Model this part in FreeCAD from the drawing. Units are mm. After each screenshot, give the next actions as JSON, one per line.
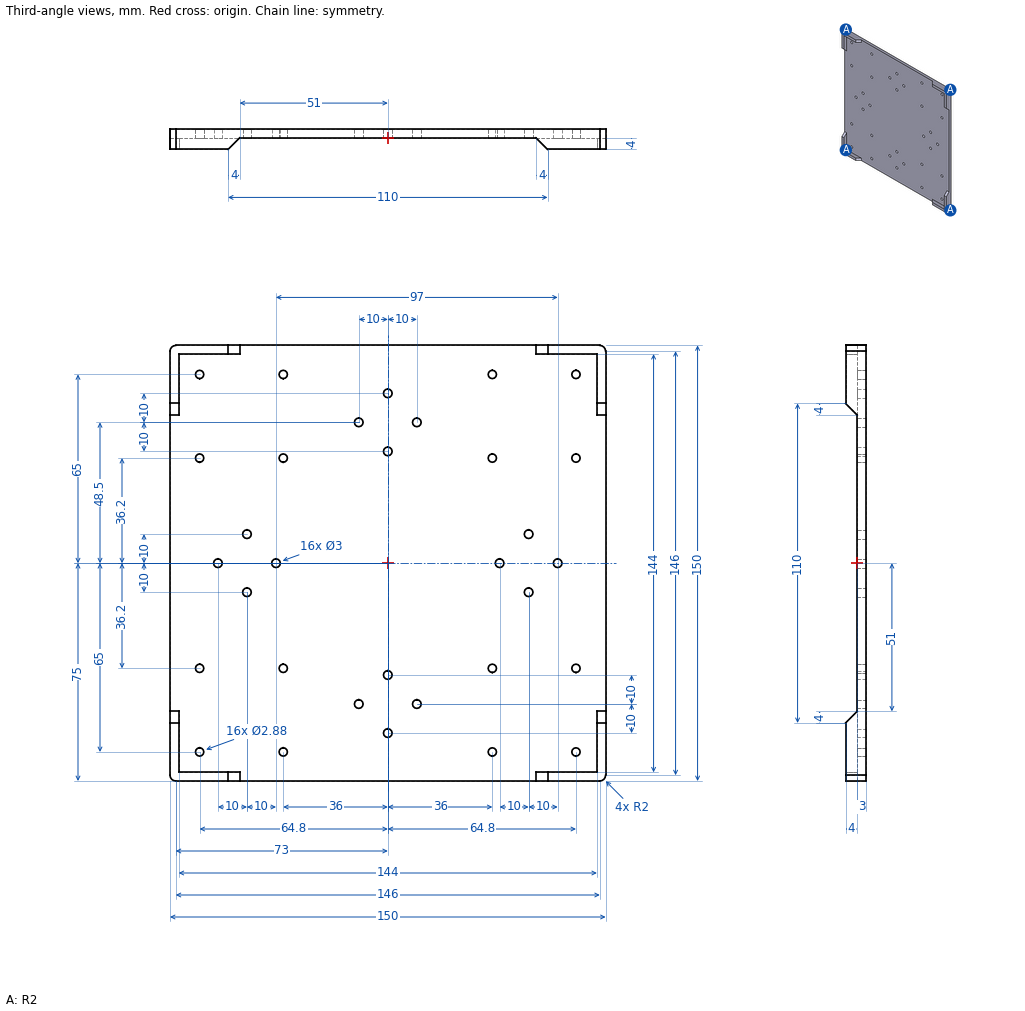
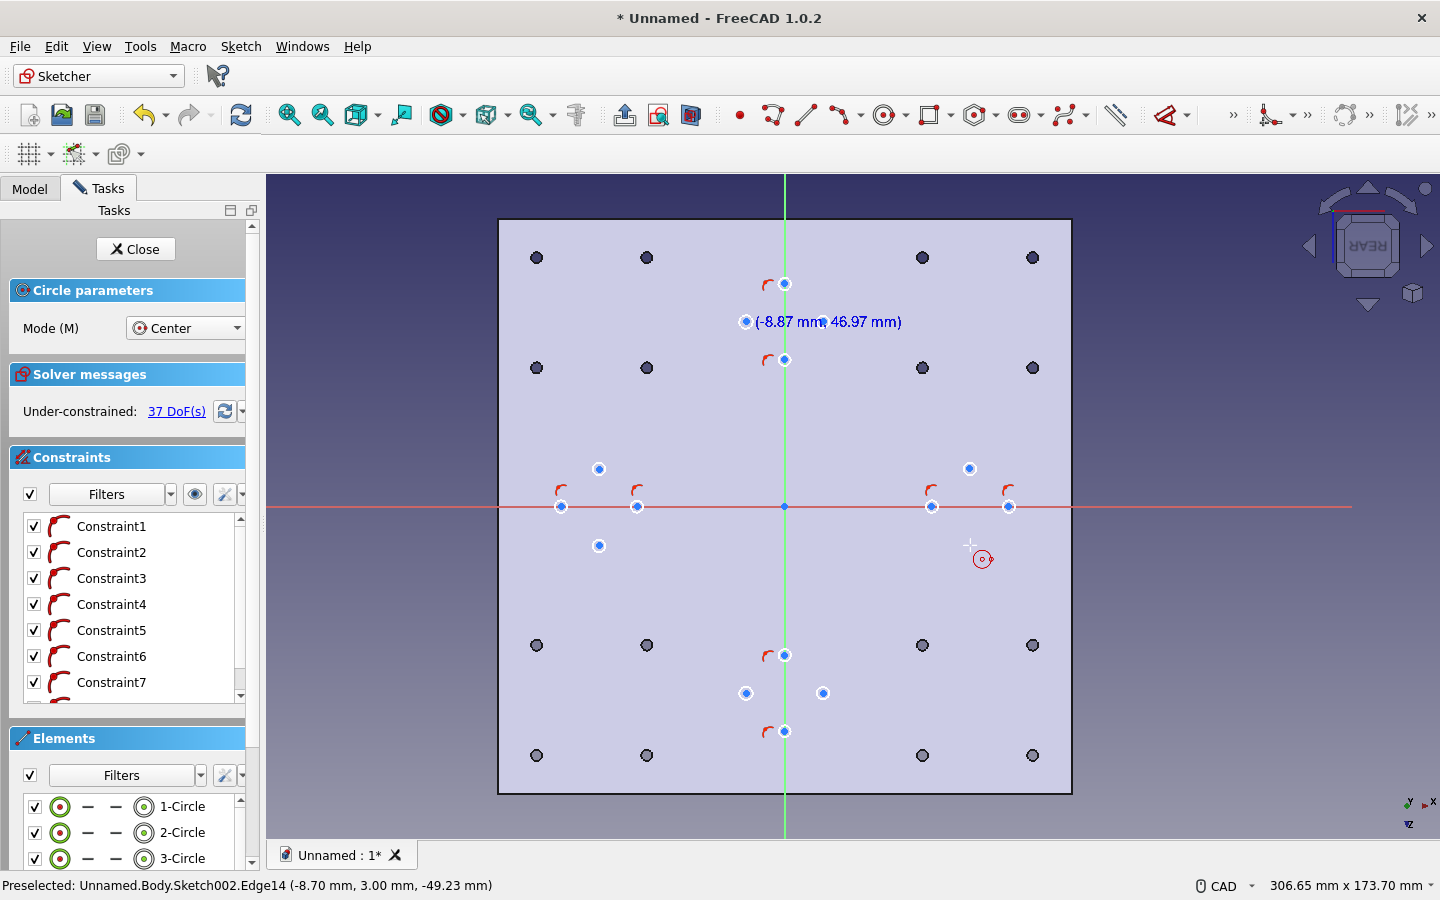
{"action": "left_click", "coordinate": [970, 545]}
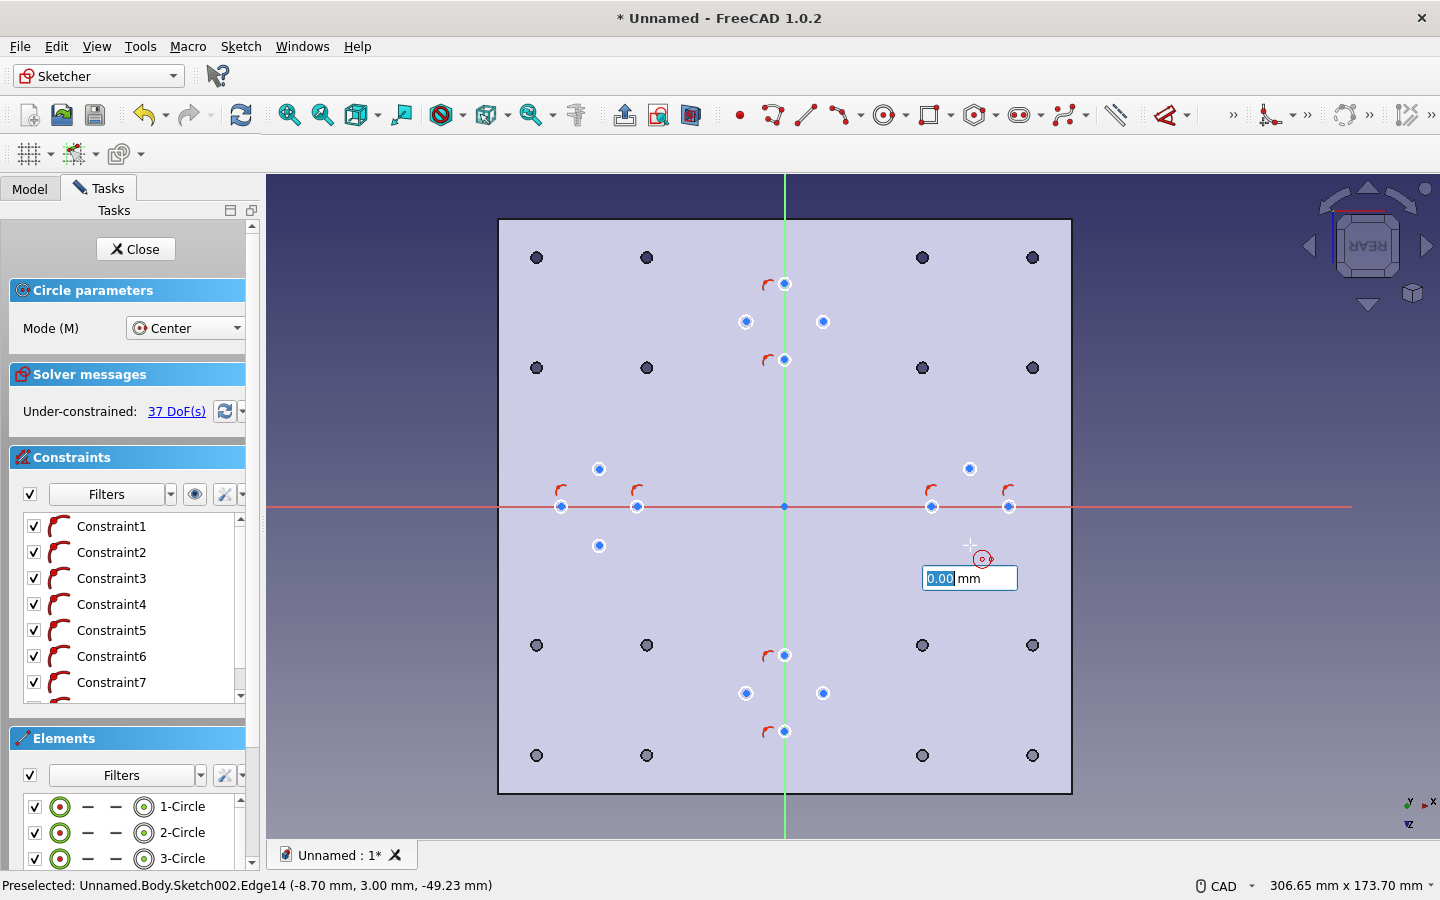
{"action": "scroll", "coordinate": [974, 541], "scroll_direction": "up", "scroll_amount": 6}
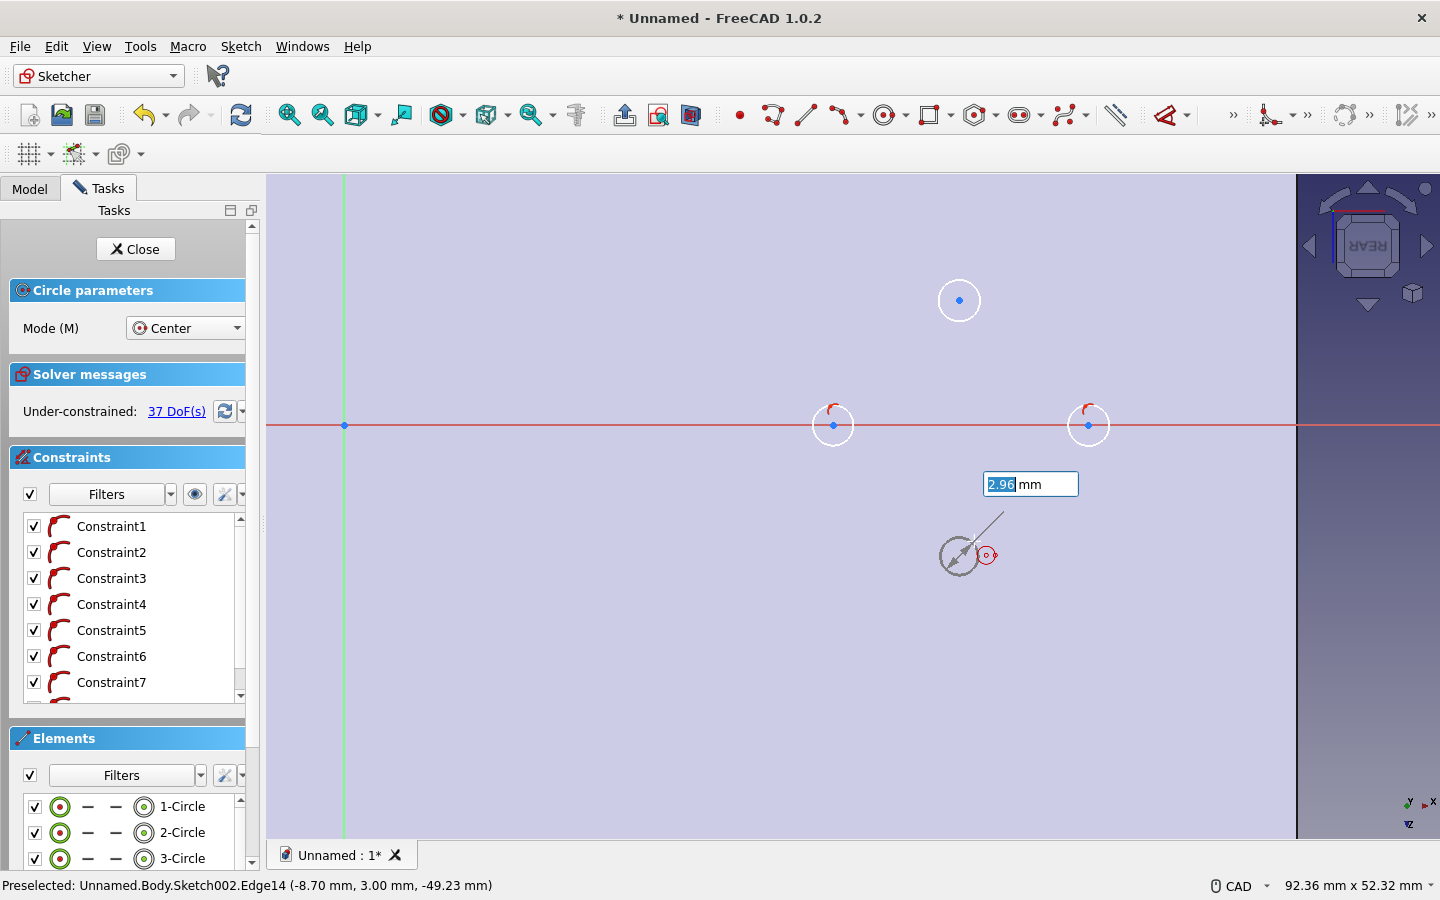
{"action": "left_click", "coordinate": [974, 539]}
{"action": "key", "text": "Escape"}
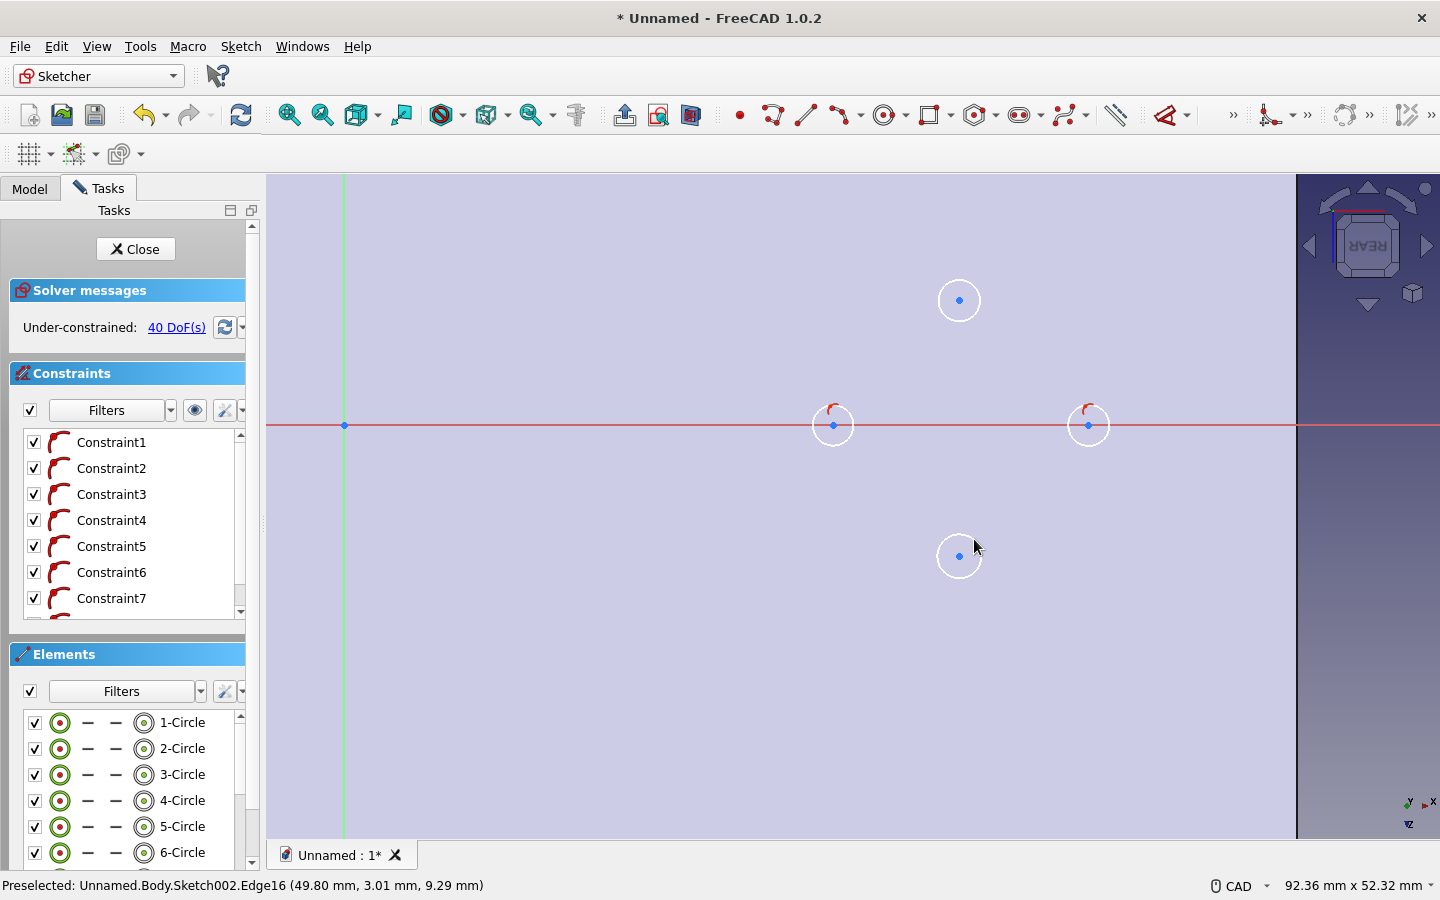
{"action": "scroll", "coordinate": [974, 541], "scroll_direction": "down", "scroll_amount": 6}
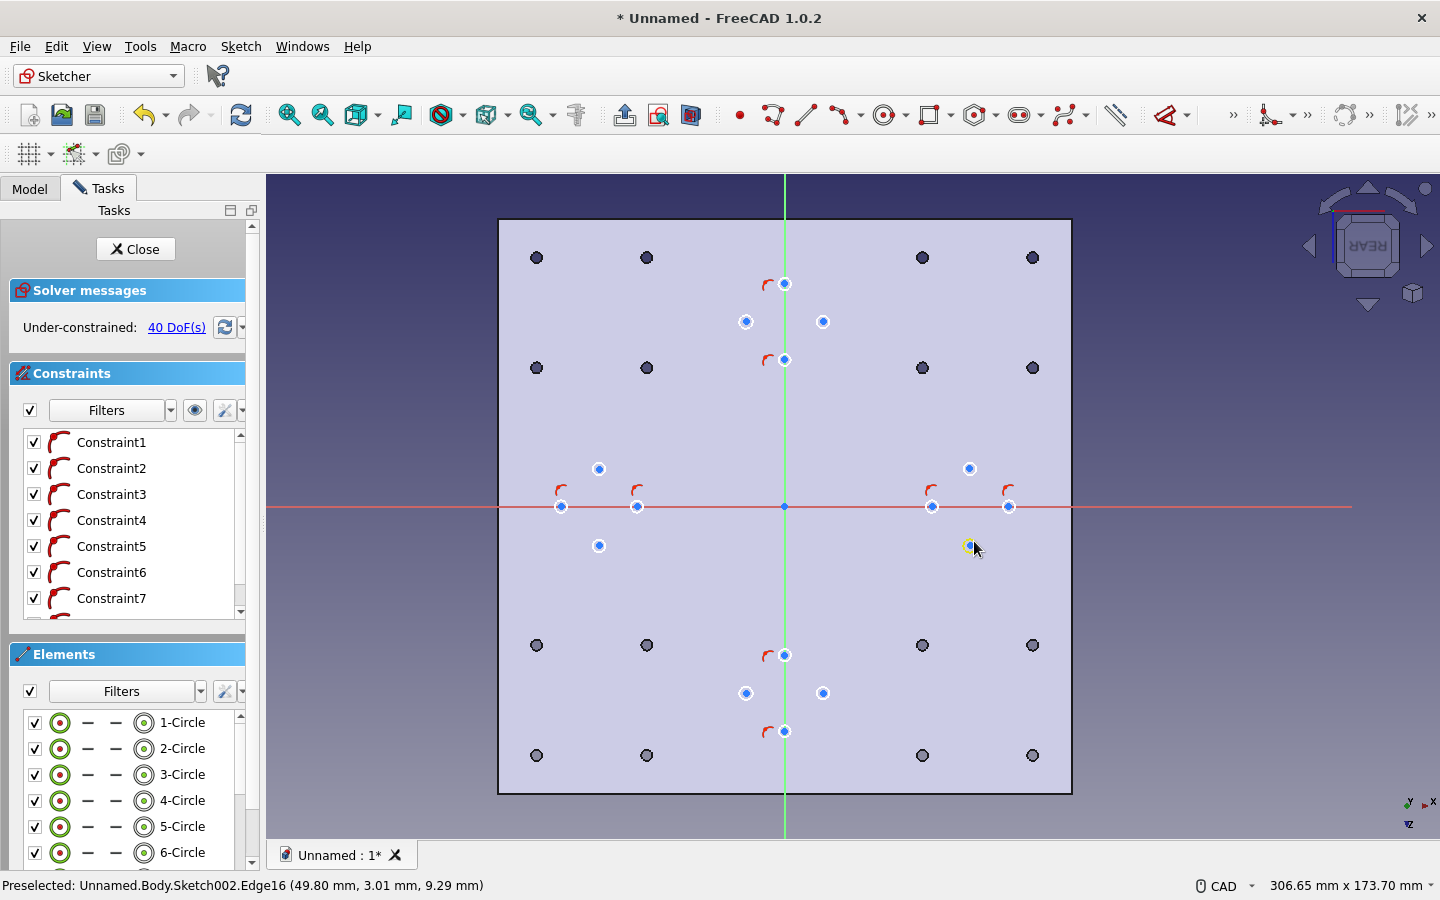
{"action": "scroll", "coordinate": [641, 502], "scroll_direction": "up", "scroll_amount": 6}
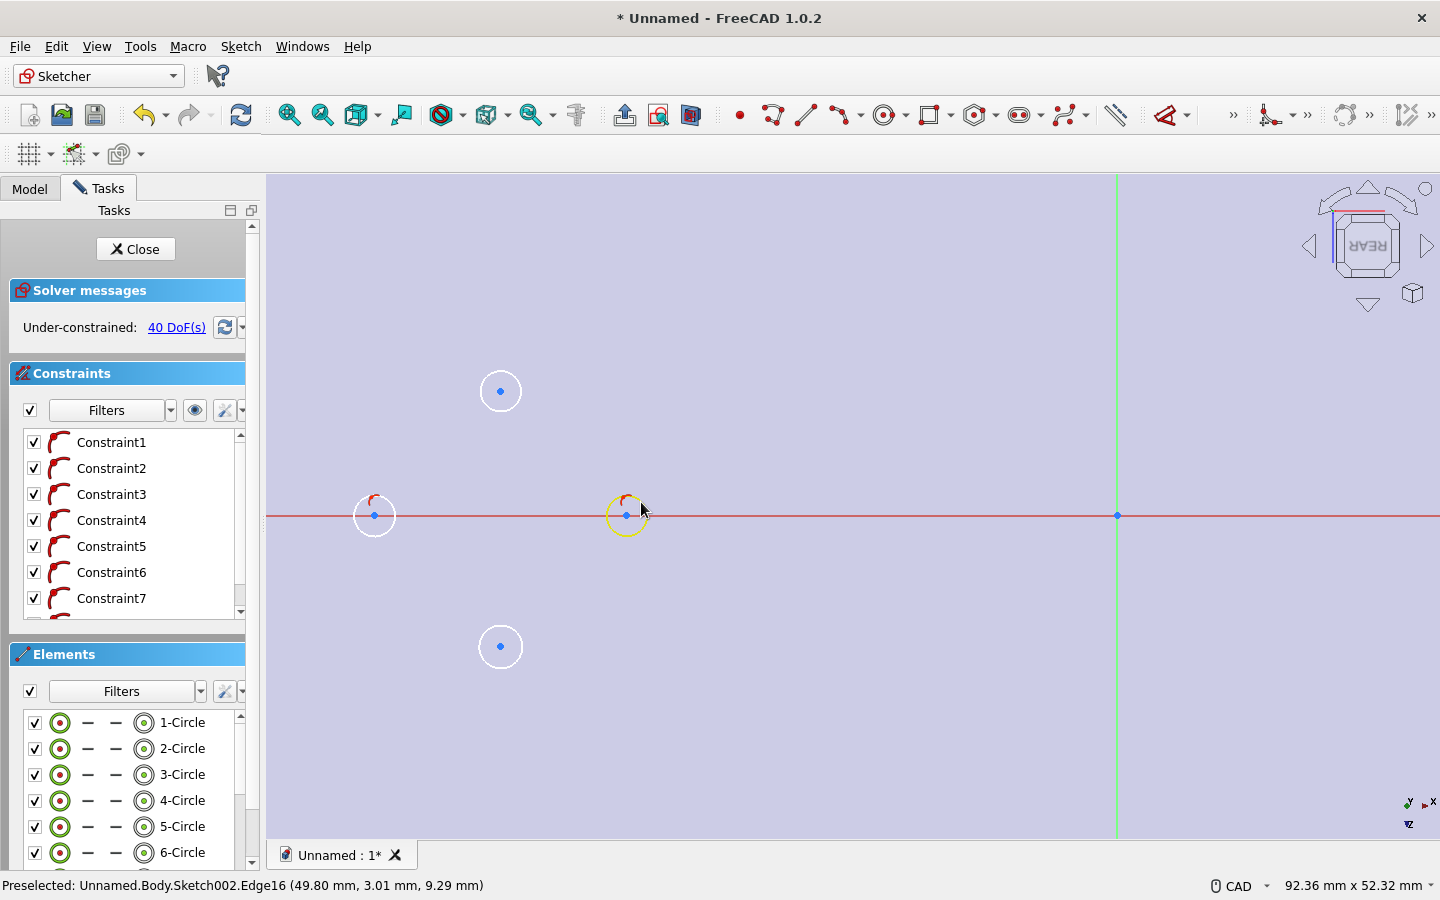
{"action": "left_click", "coordinate": [641, 502]}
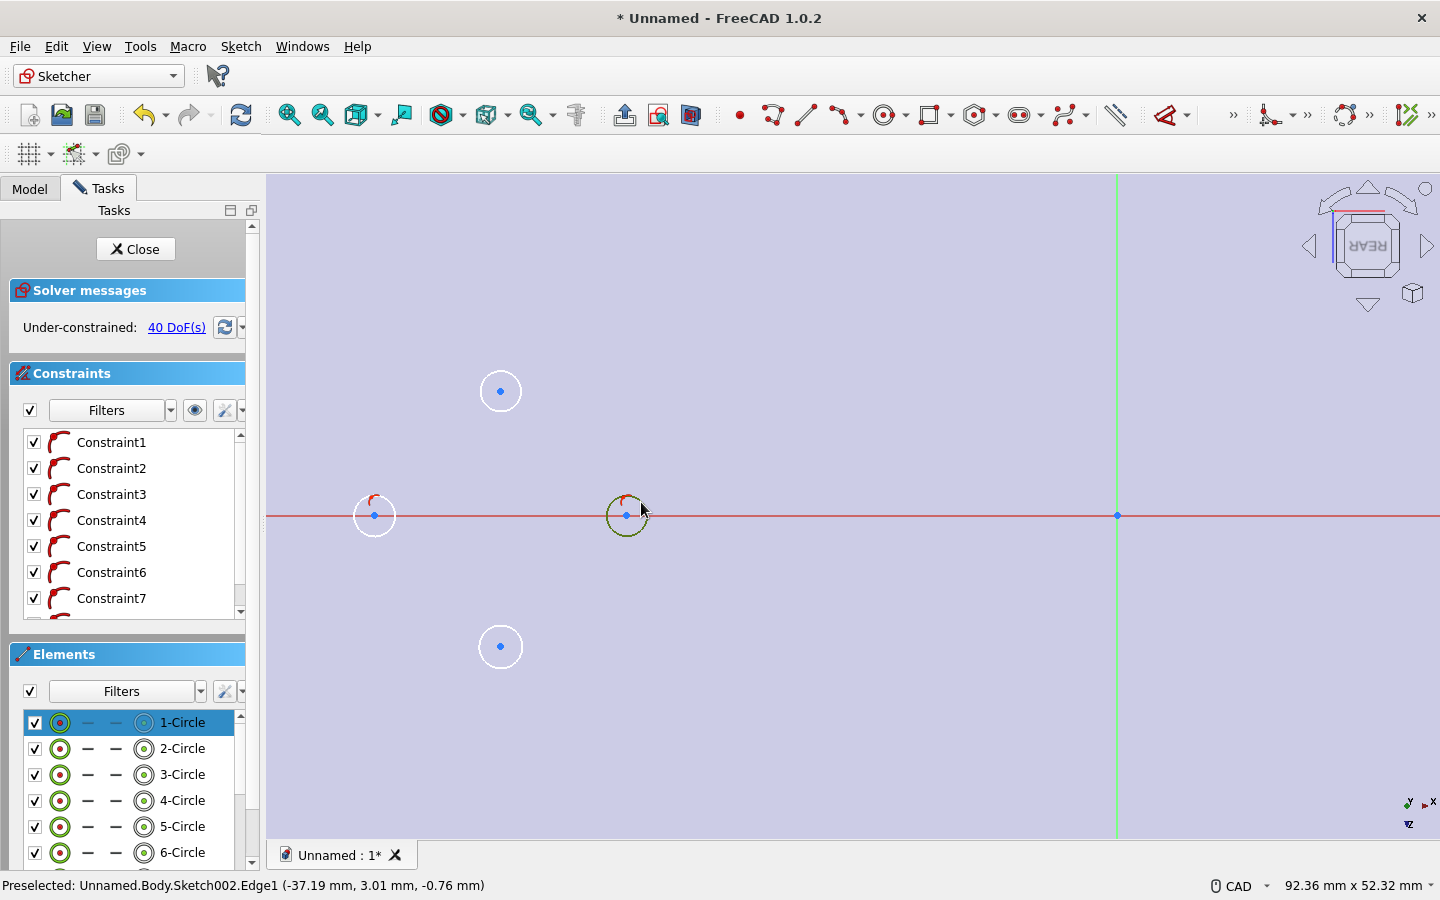
{"action": "left_click", "coordinate": [515, 377]}